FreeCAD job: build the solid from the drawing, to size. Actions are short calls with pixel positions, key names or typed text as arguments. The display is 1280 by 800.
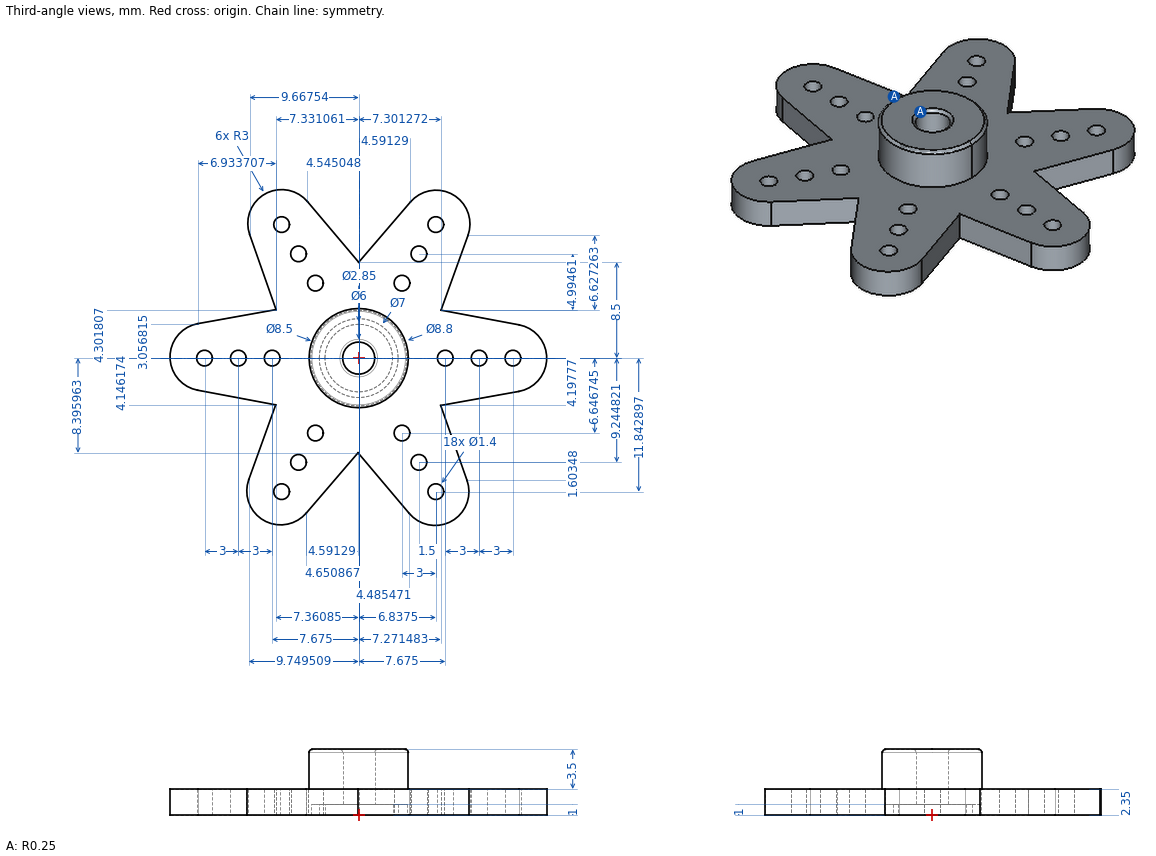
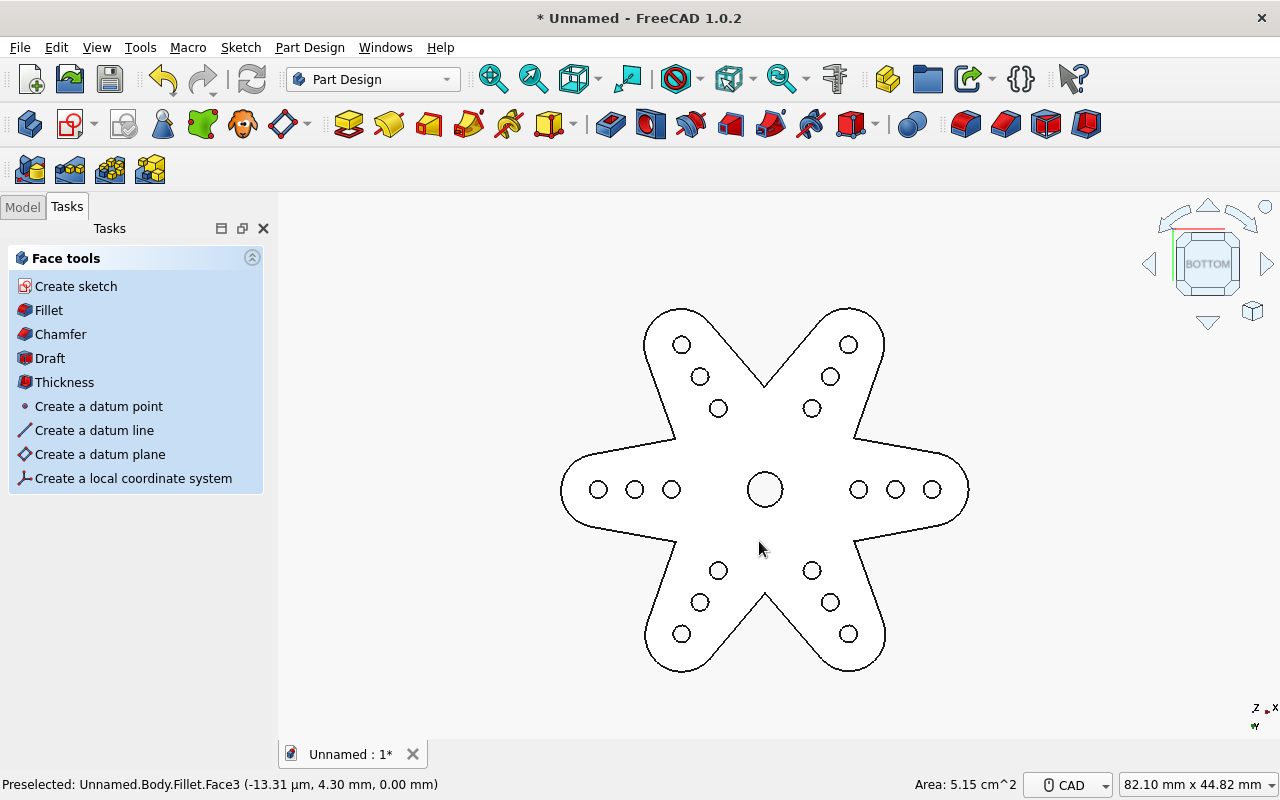
click(70, 124)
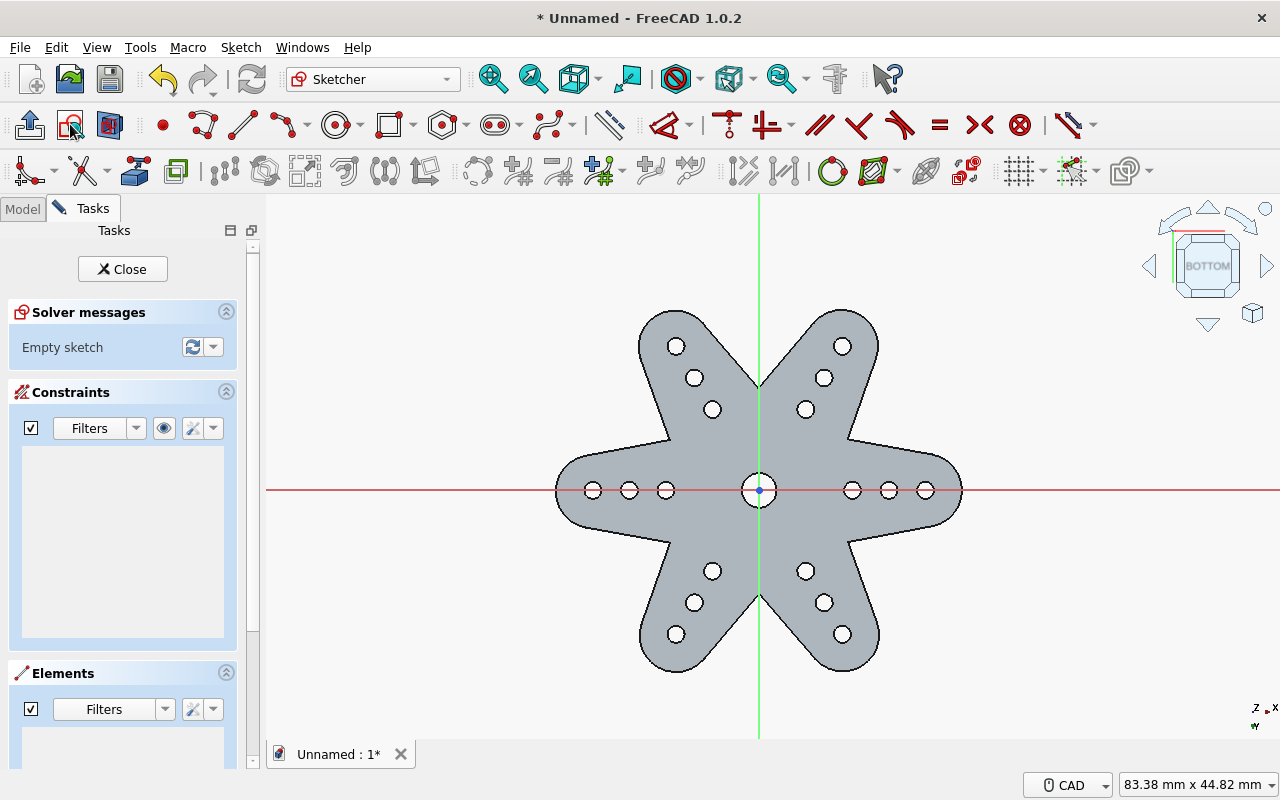
scroll(783, 501, up, 6)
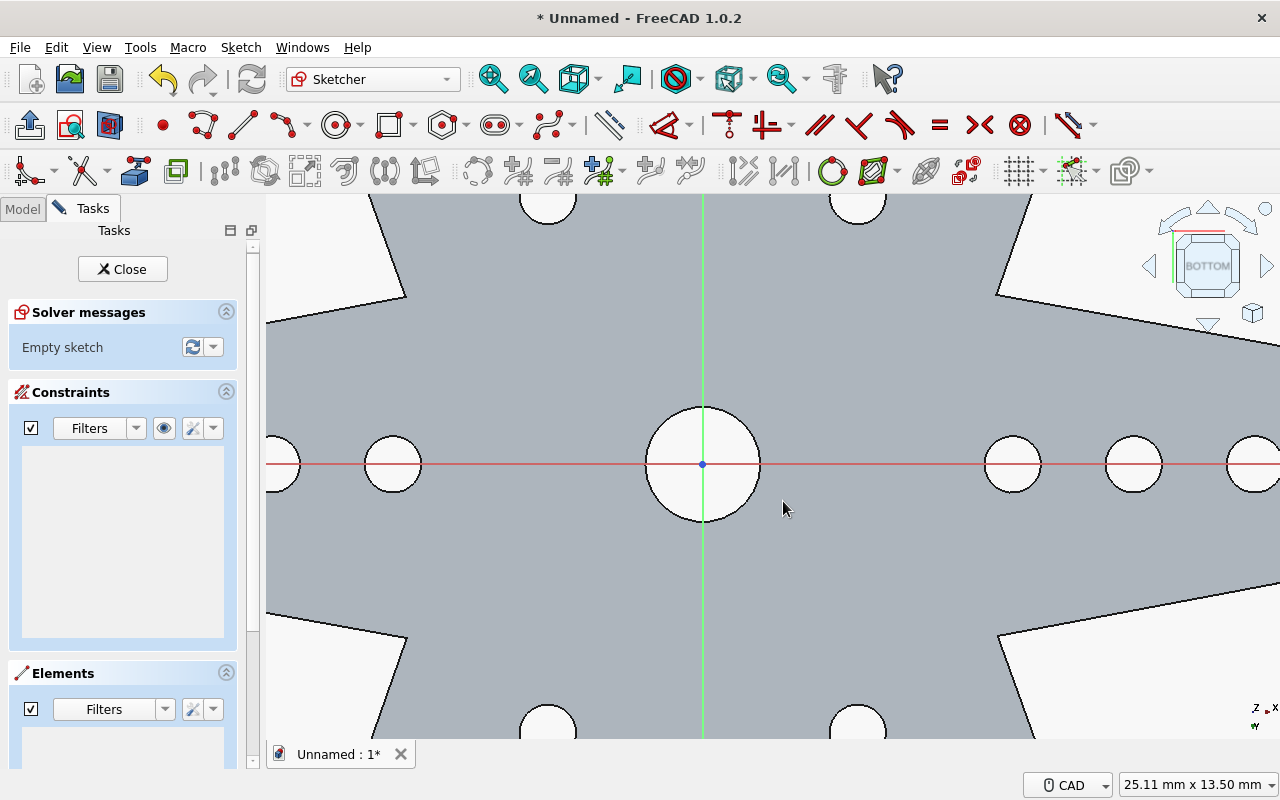
click(336, 126)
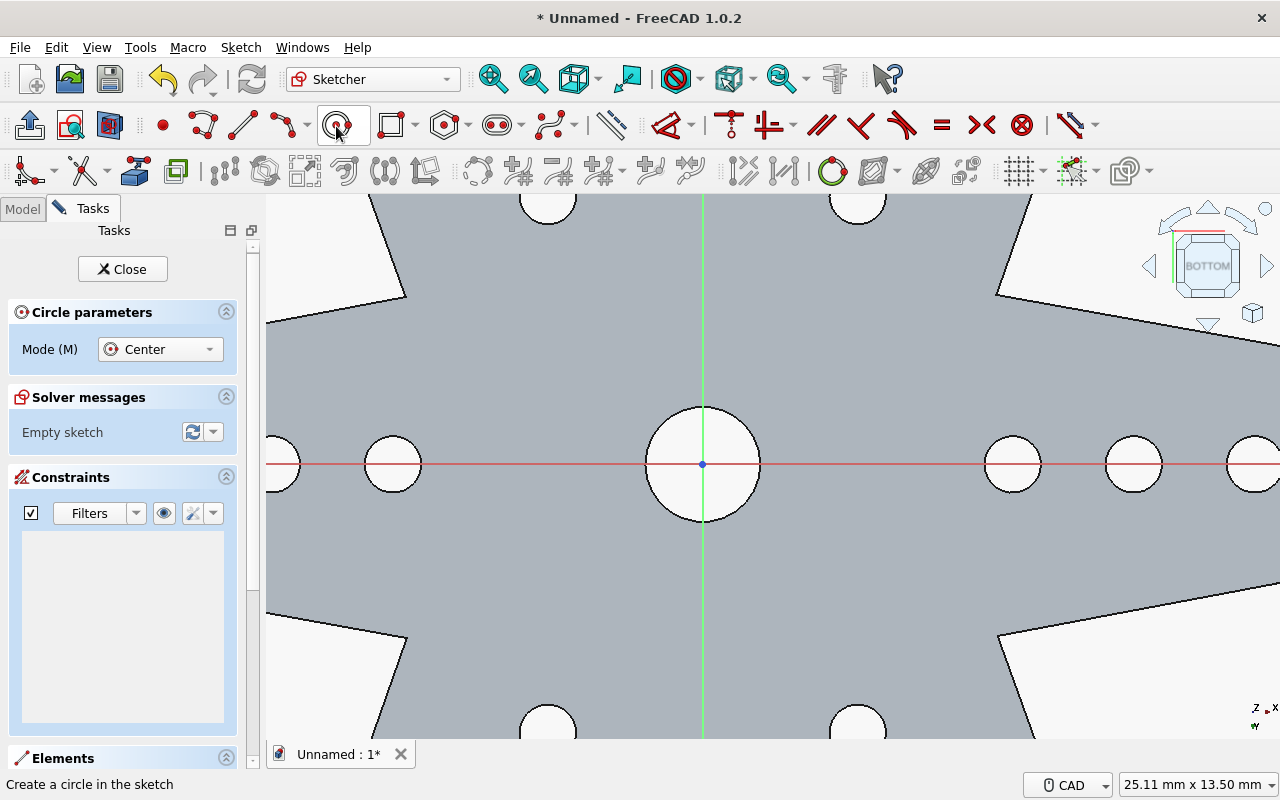
click(703, 464)
click(824, 343)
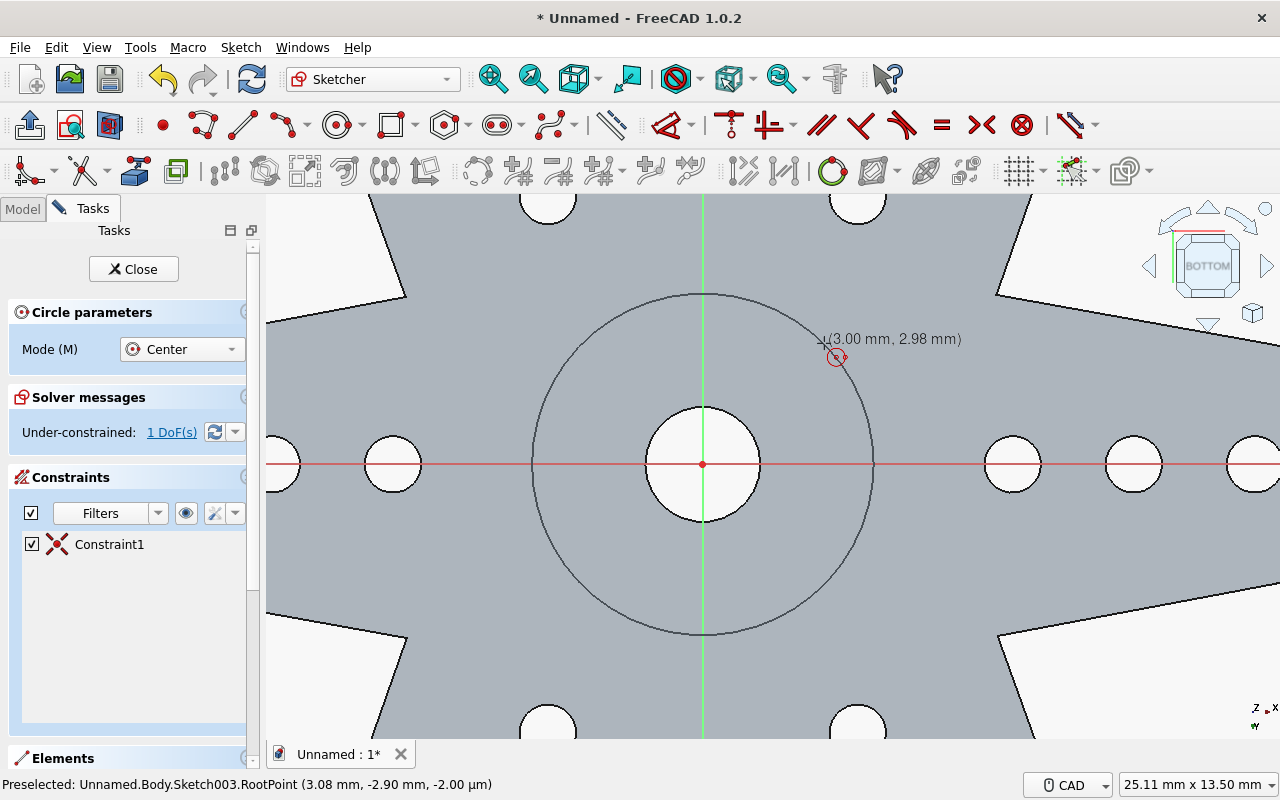
click(703, 464)
click(803, 364)
key(Escape)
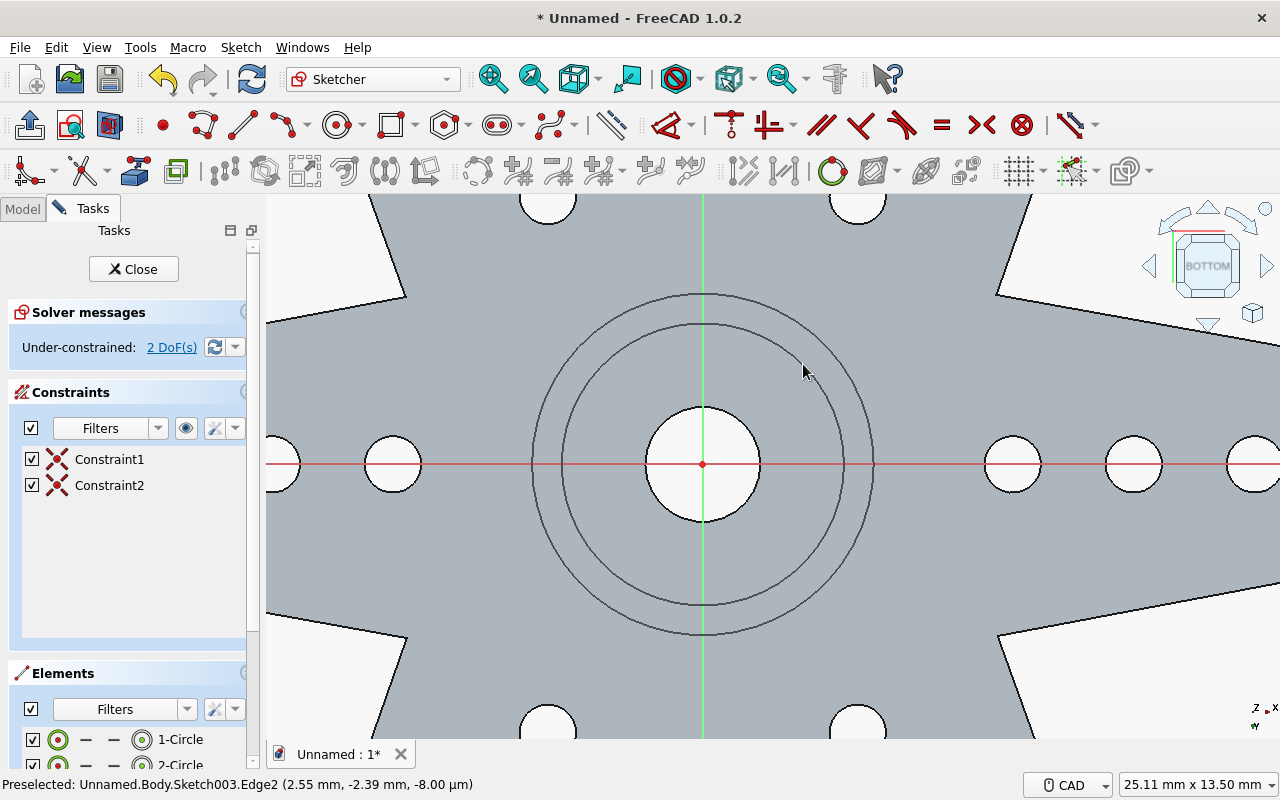
click(666, 126)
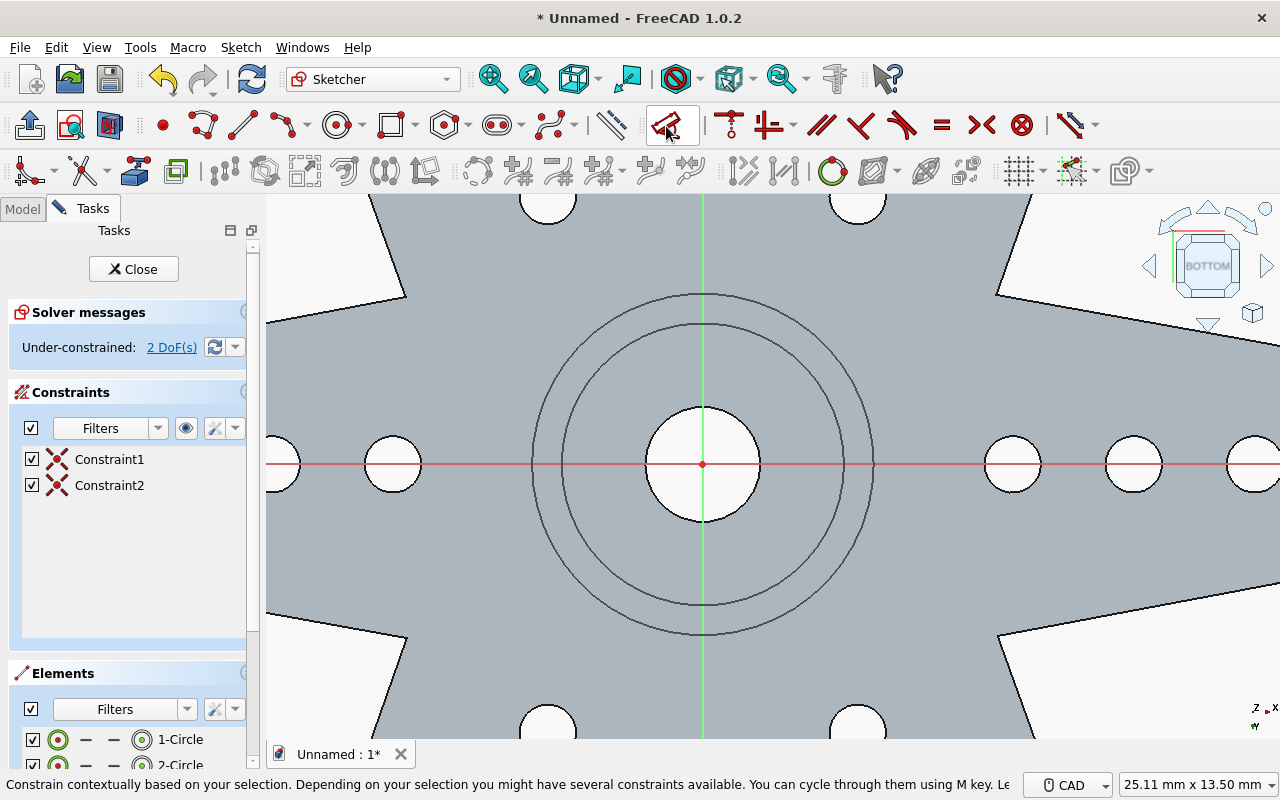
click(823, 343)
click(846, 320)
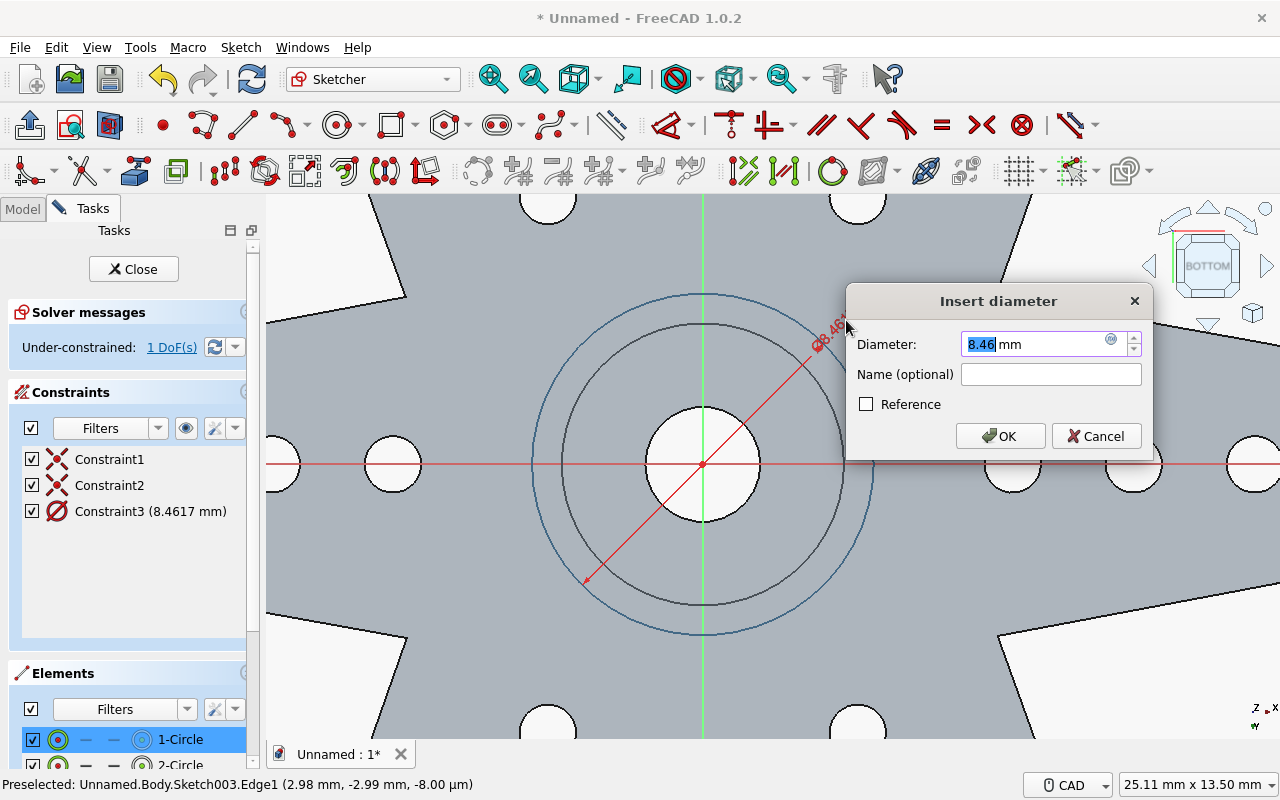
text(8.5)
key(Return)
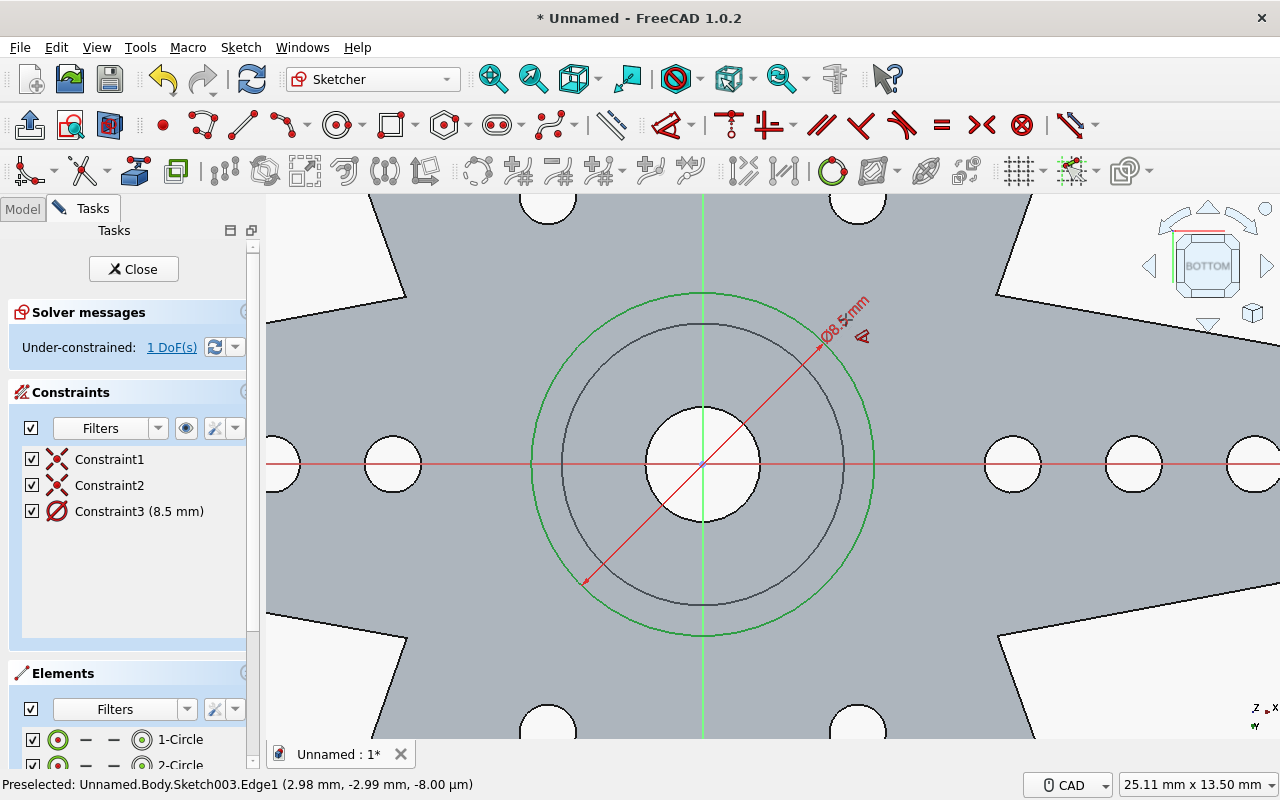
click(802, 364)
click(891, 408)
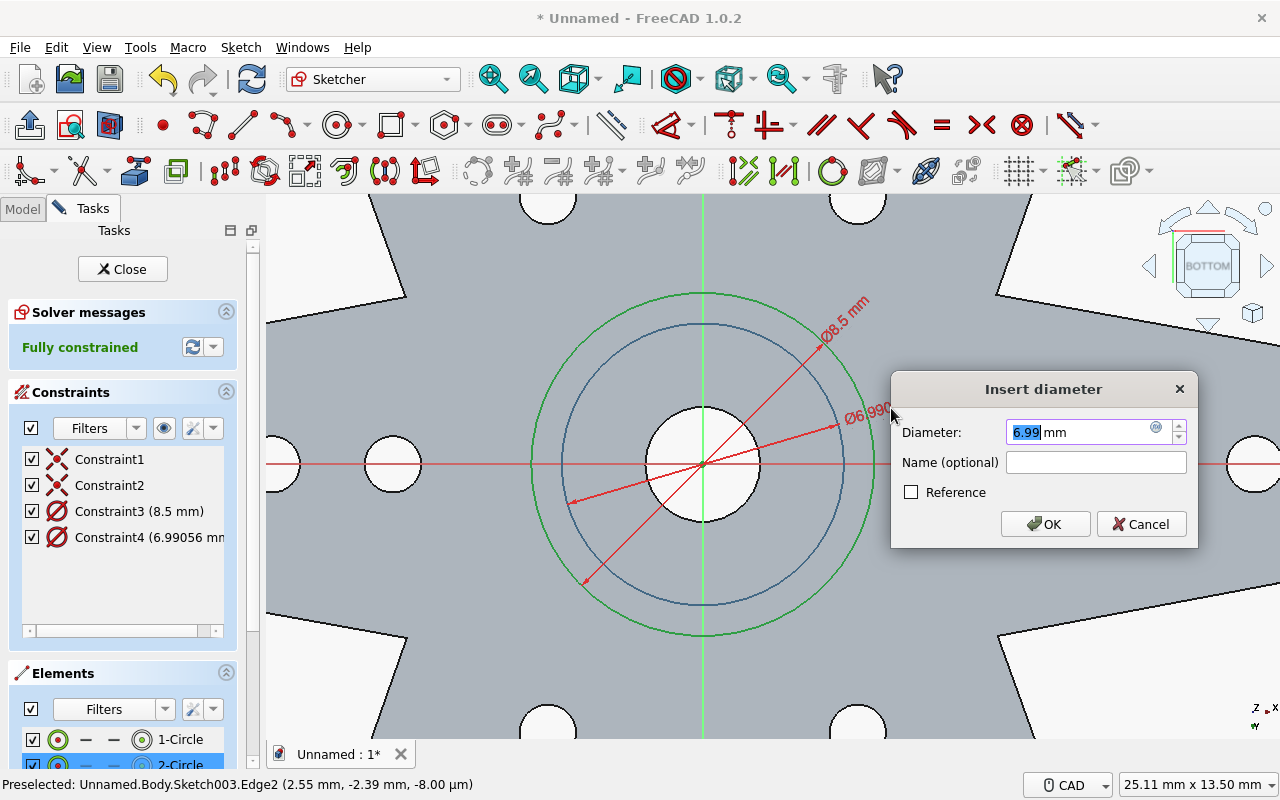
text(7)
key(Return)
key(Escape)